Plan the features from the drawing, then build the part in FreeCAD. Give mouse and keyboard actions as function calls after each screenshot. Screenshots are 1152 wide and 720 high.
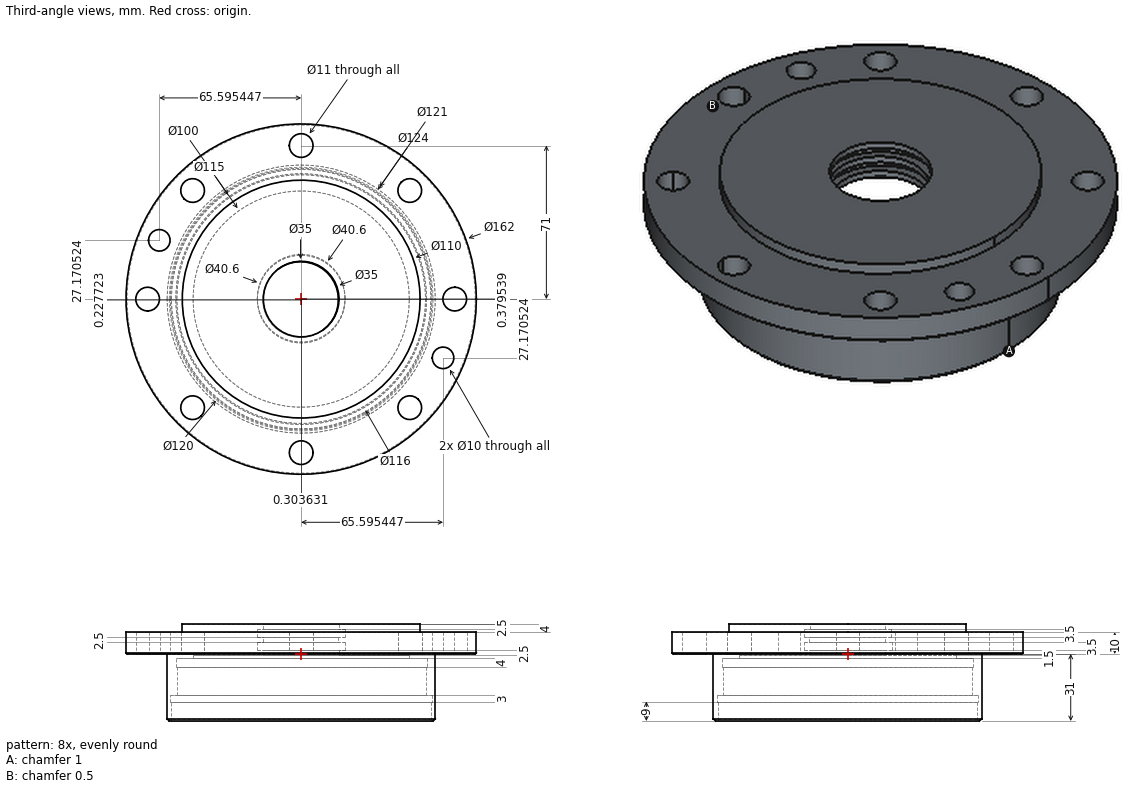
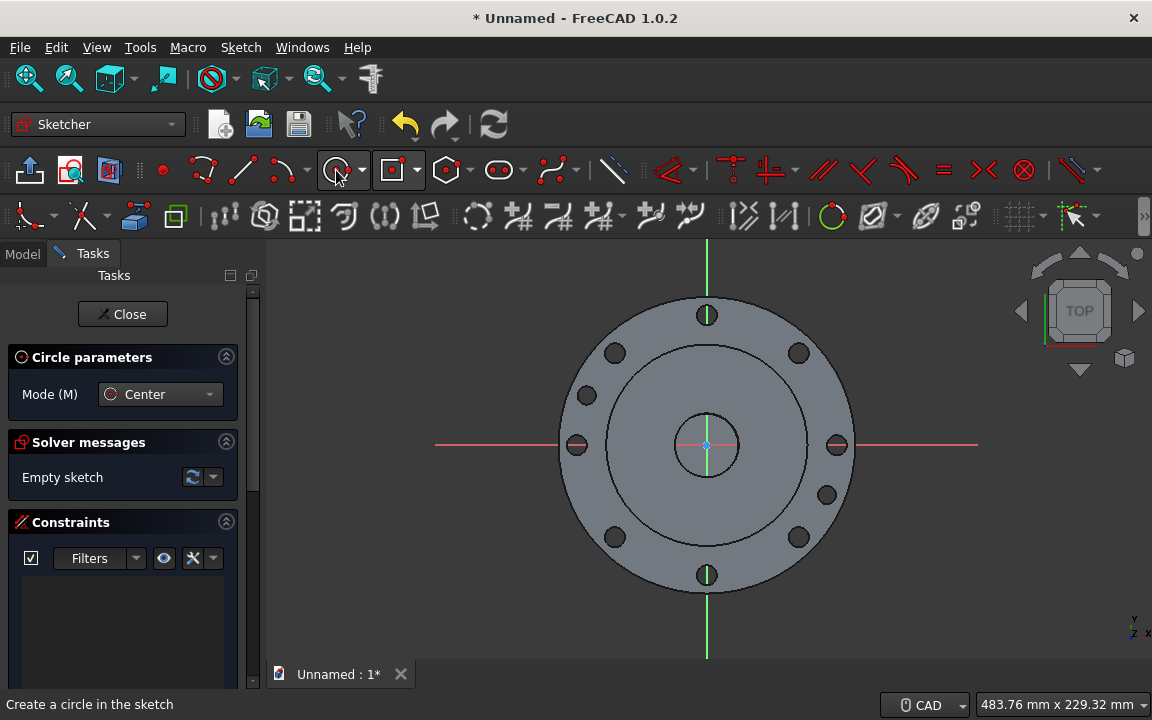
click(707, 445)
click(782, 370)
key(Escape)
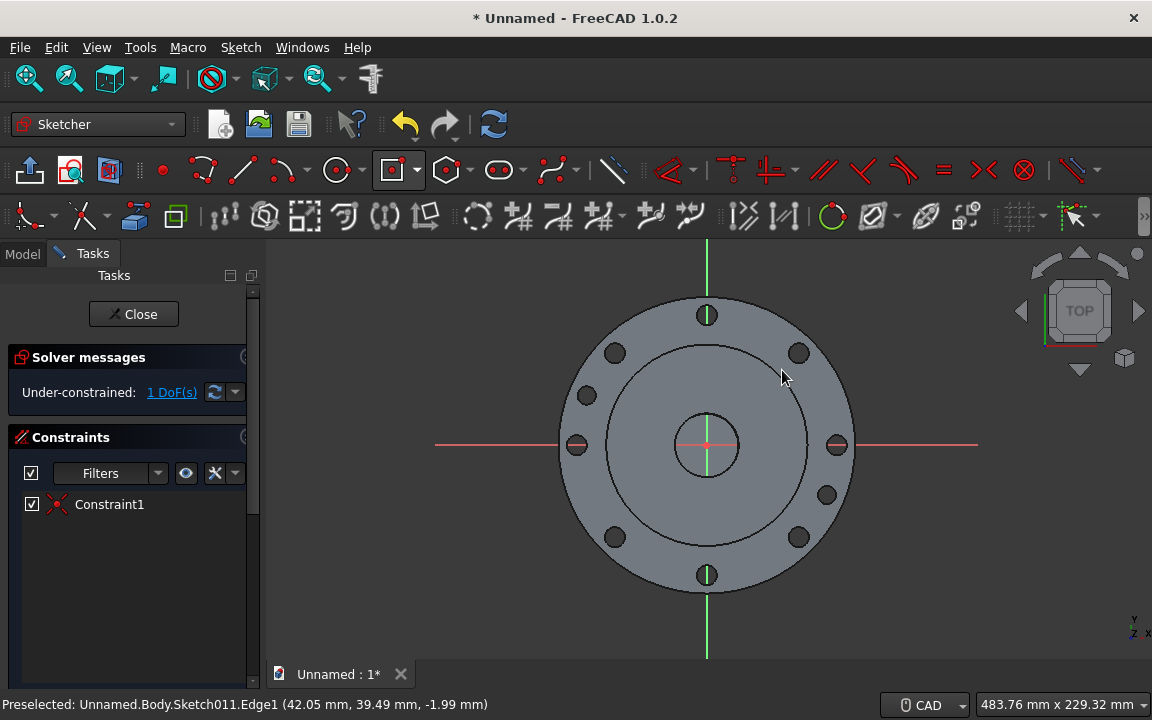
click(668, 170)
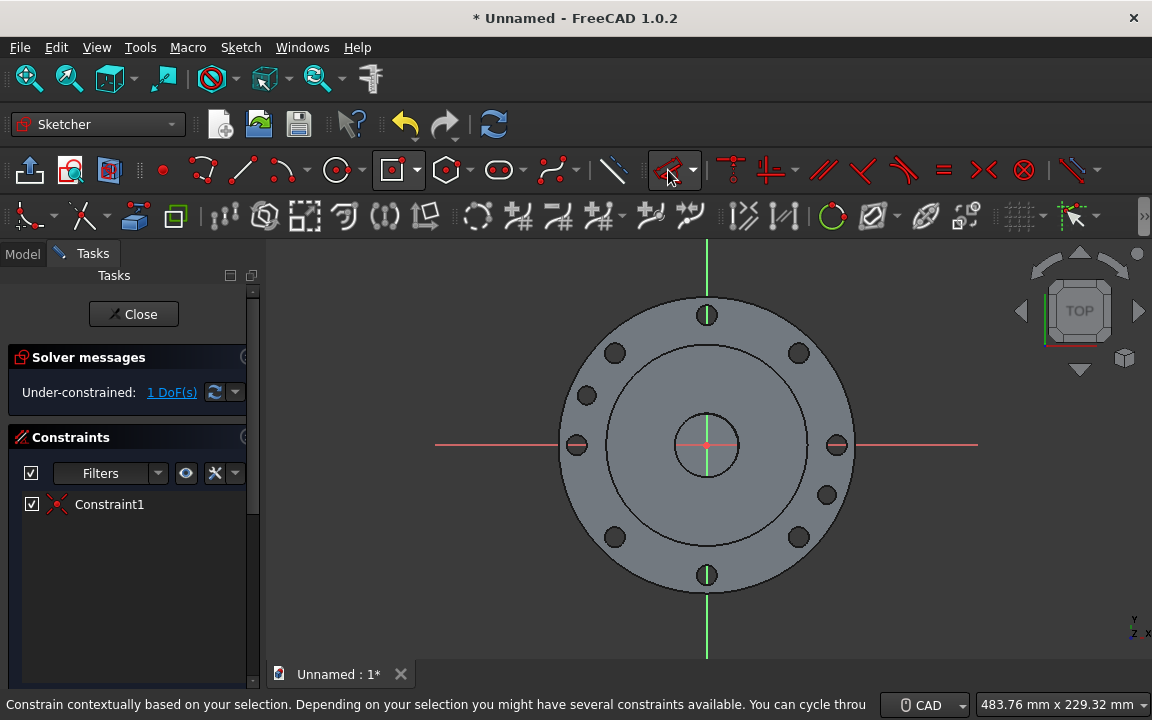
click(781, 370)
click(803, 347)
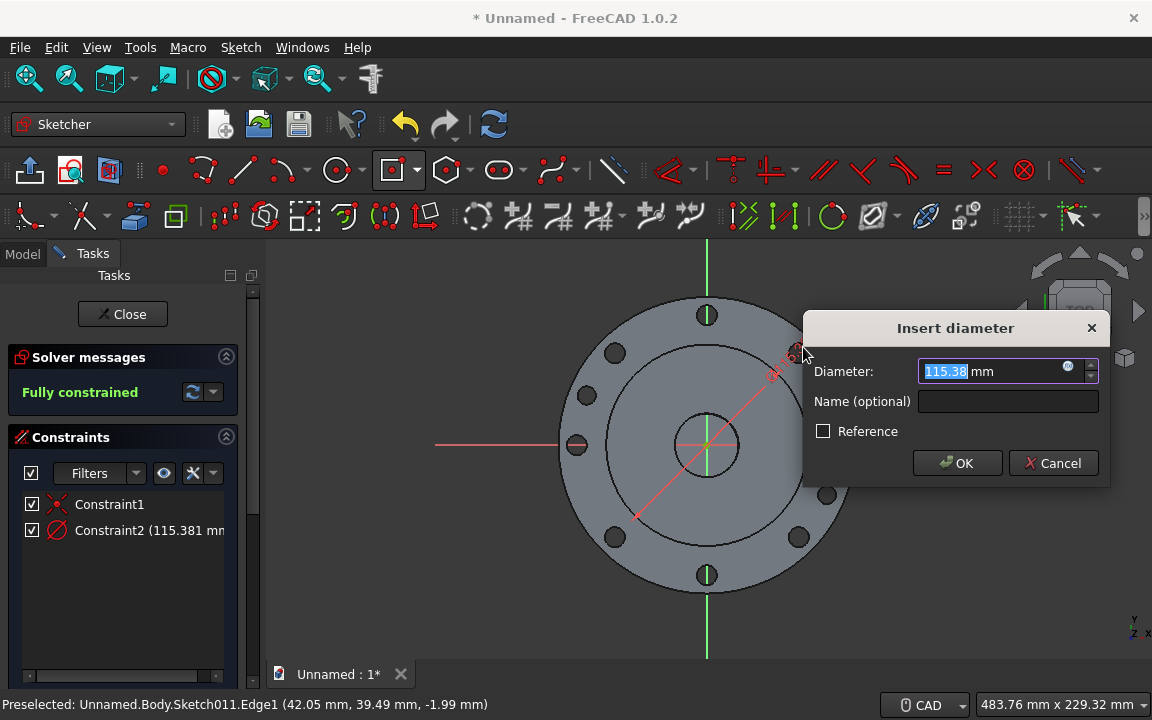
text(116)
key(Return)
key(Escape)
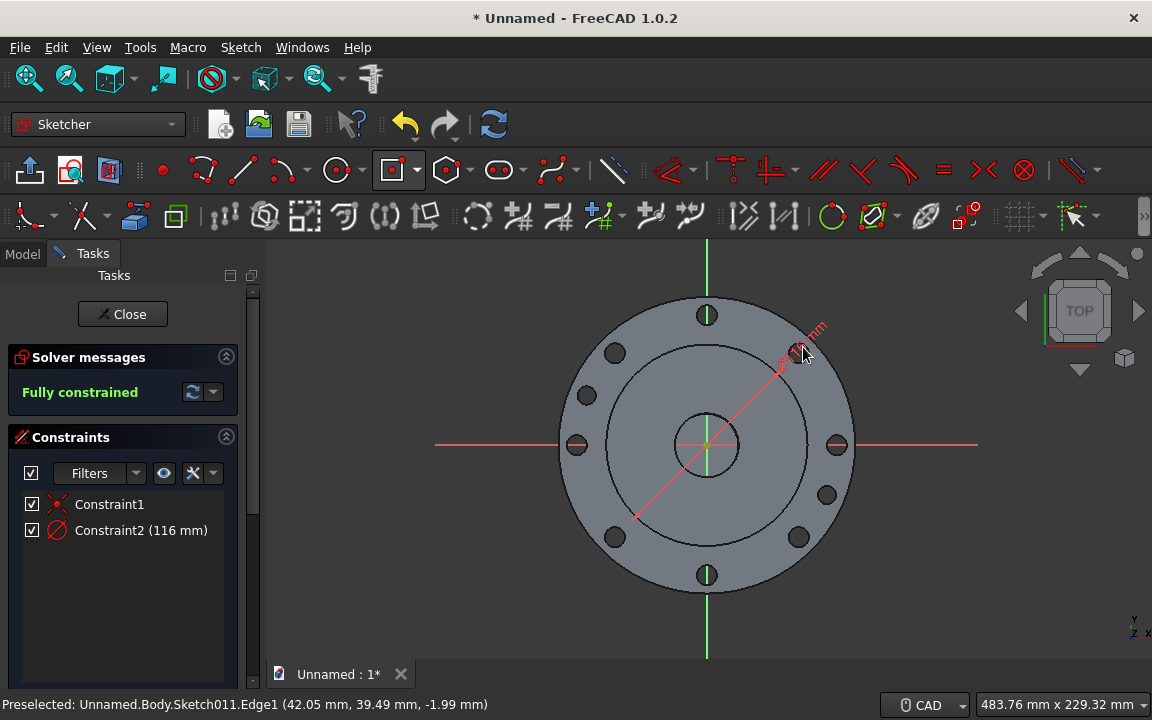
click(123, 314)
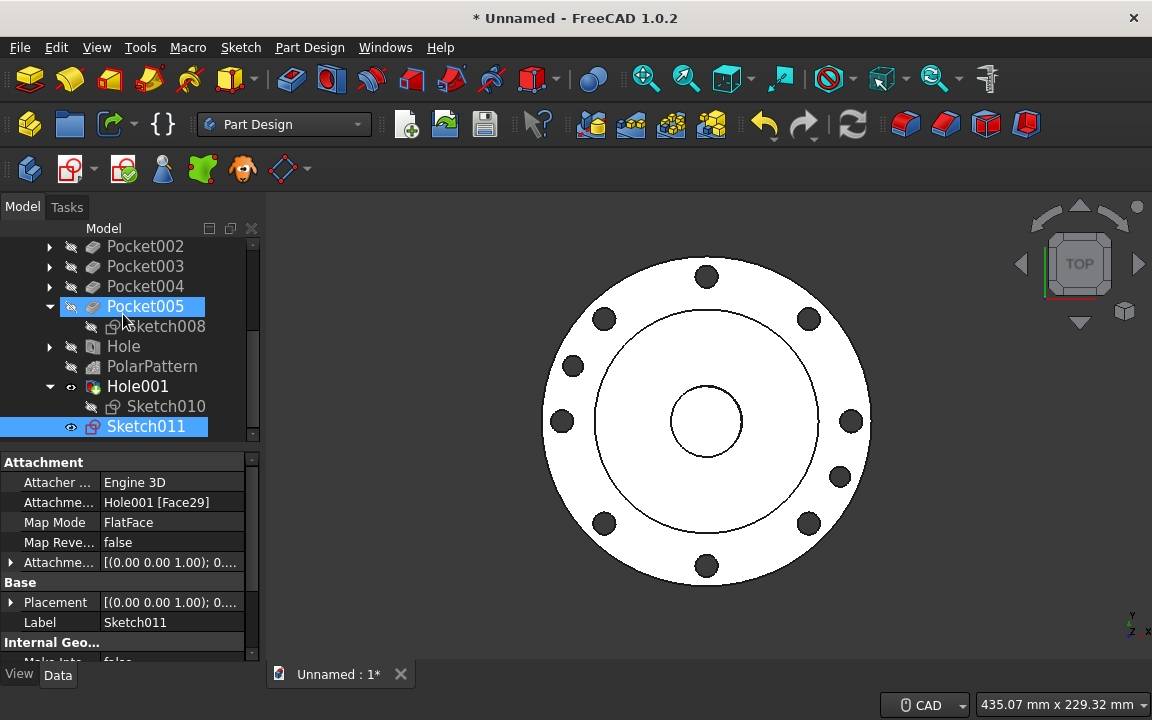
click(292, 80)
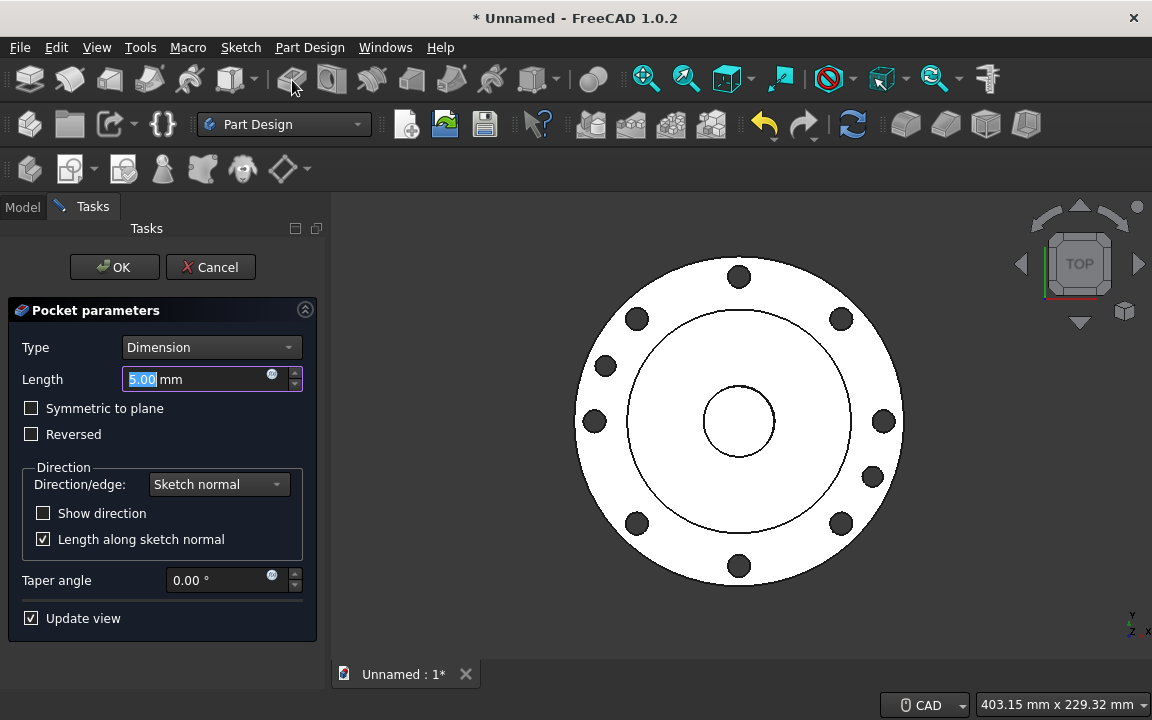
text(4)
key(Tab)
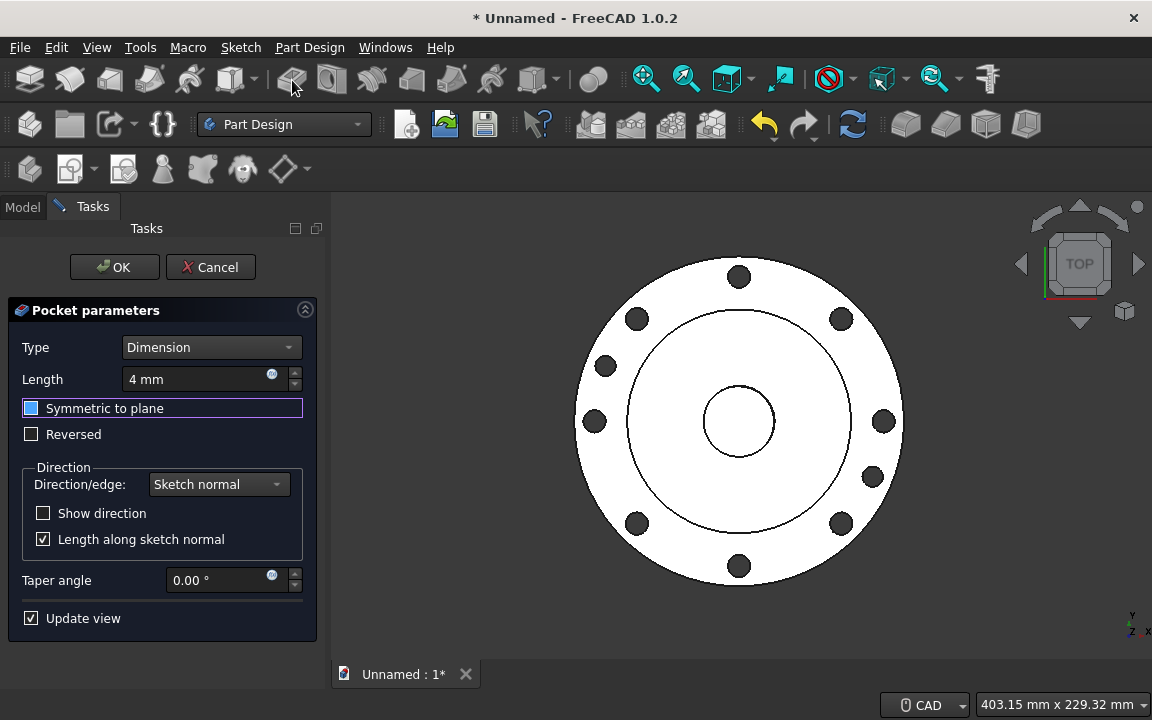
click(115, 267)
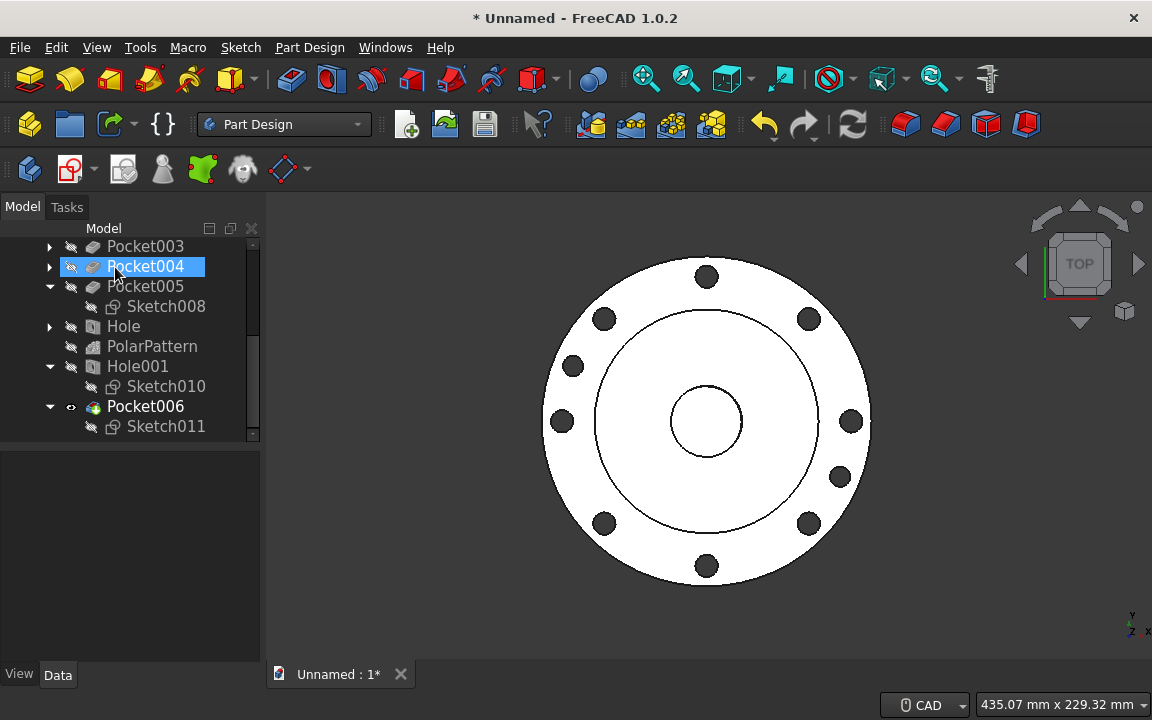
key(5)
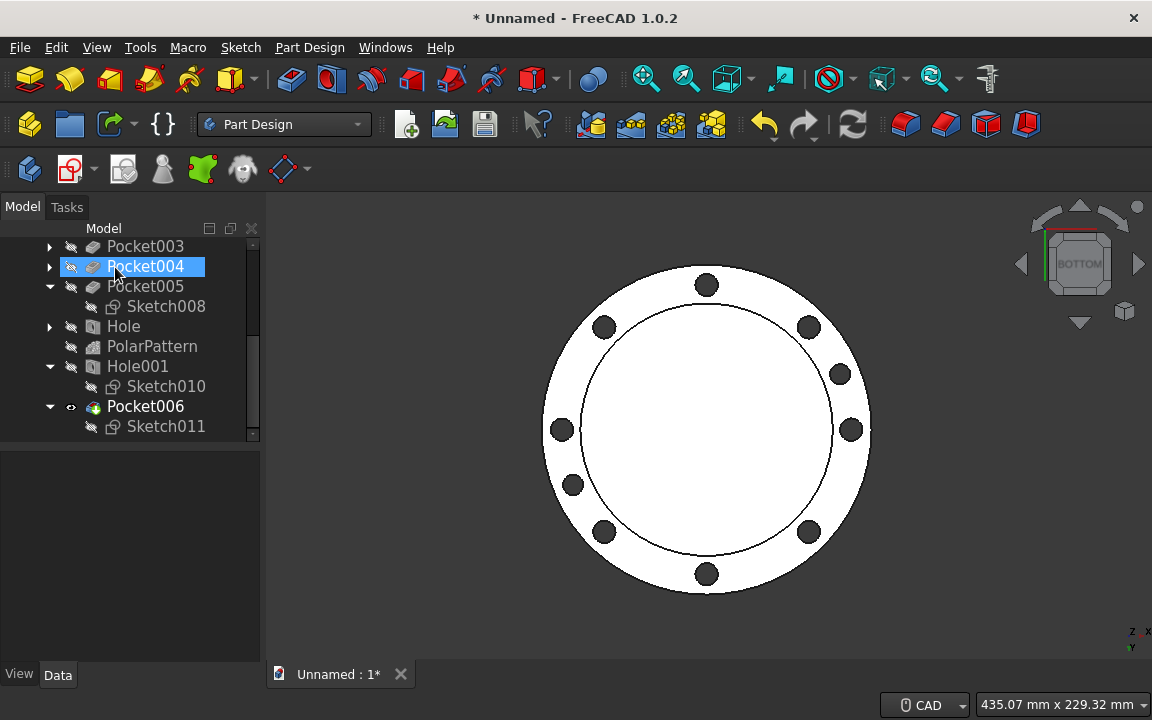
click(707, 429)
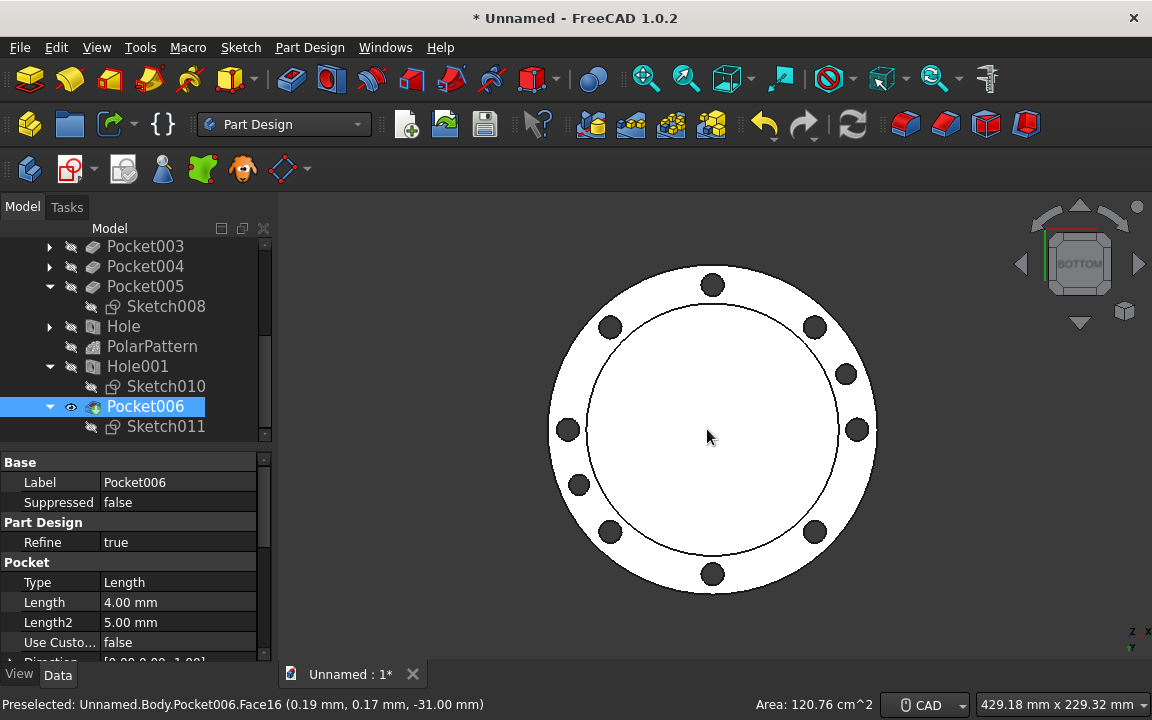
click(70, 170)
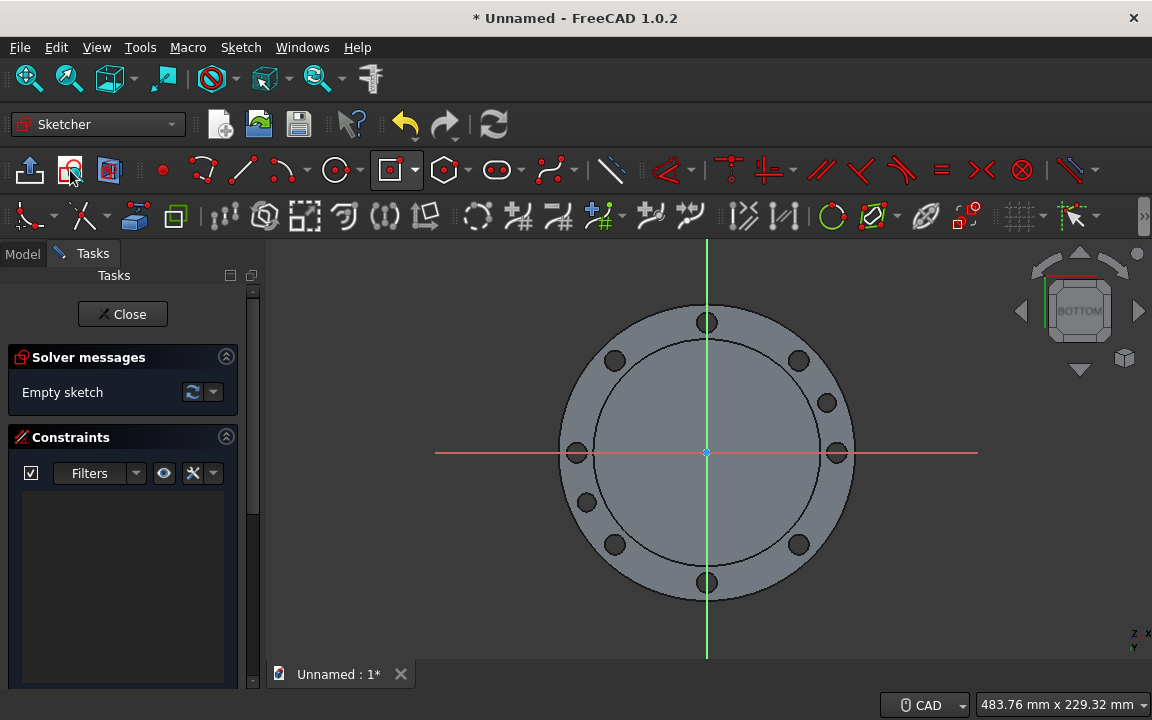
key(g)
key(c)